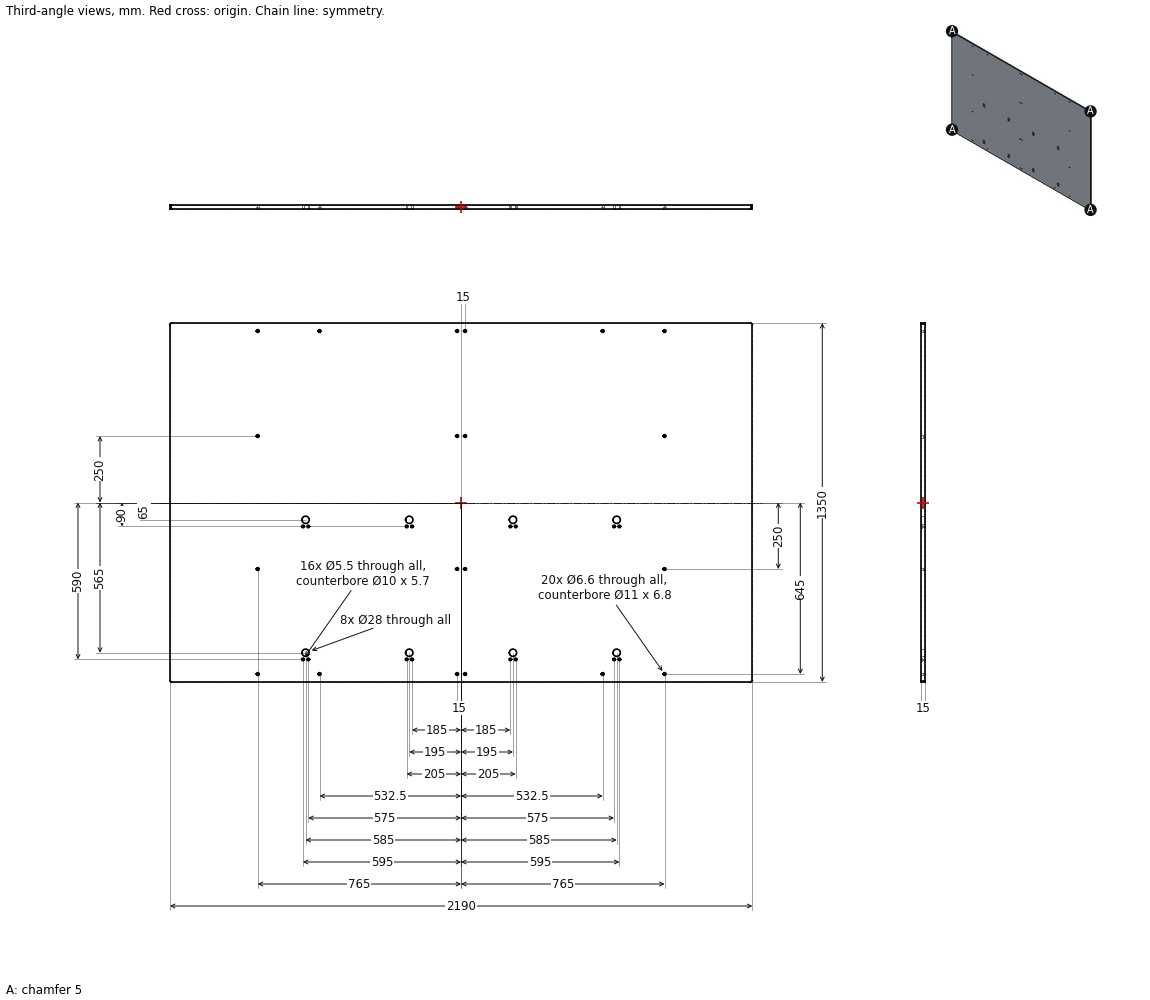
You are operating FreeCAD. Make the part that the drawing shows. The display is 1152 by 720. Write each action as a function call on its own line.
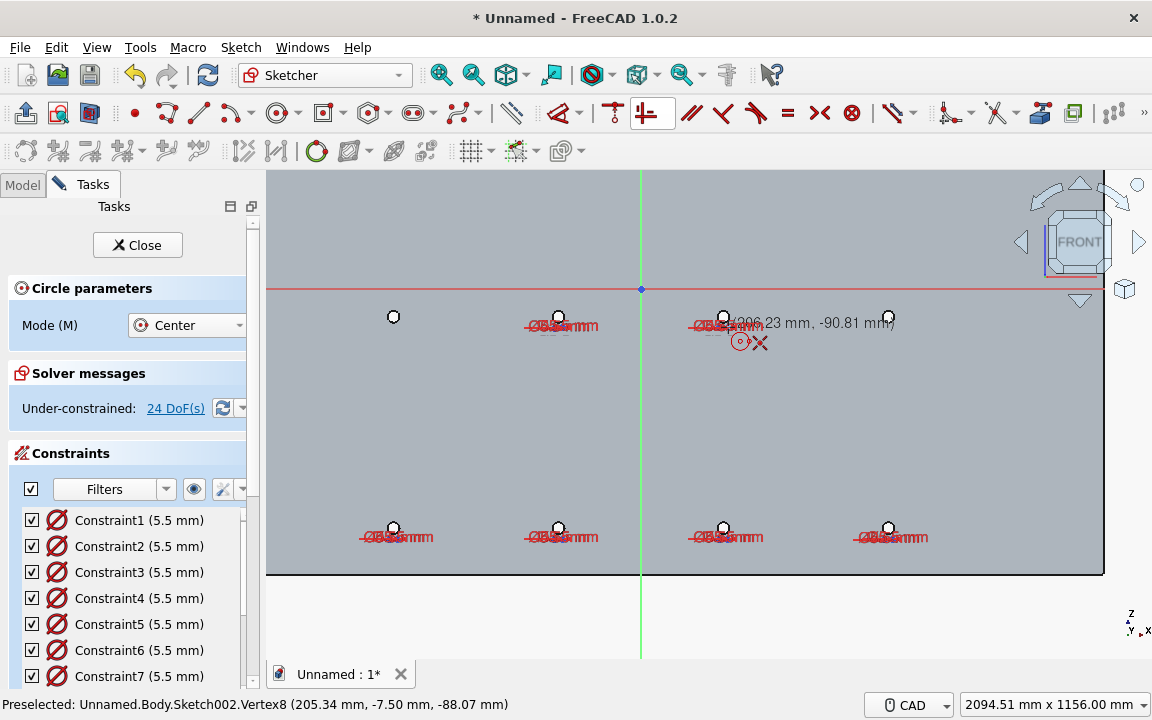
scroll(884, 327, up, 15)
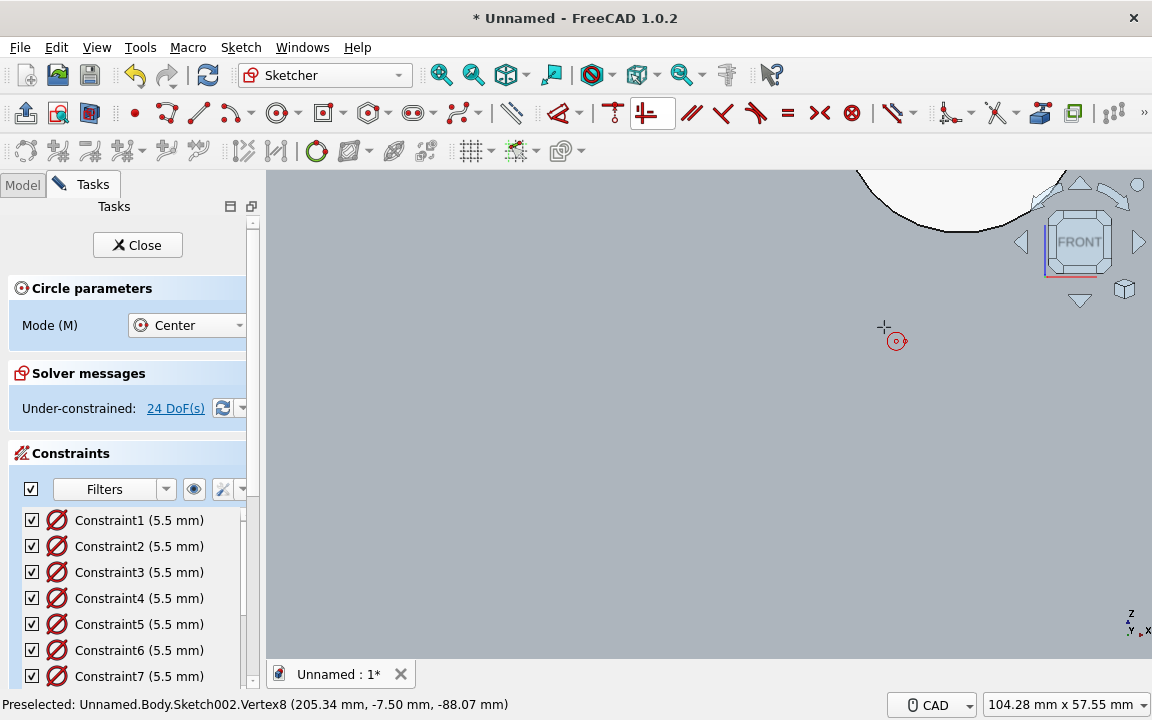
scroll(884, 327, down, 15)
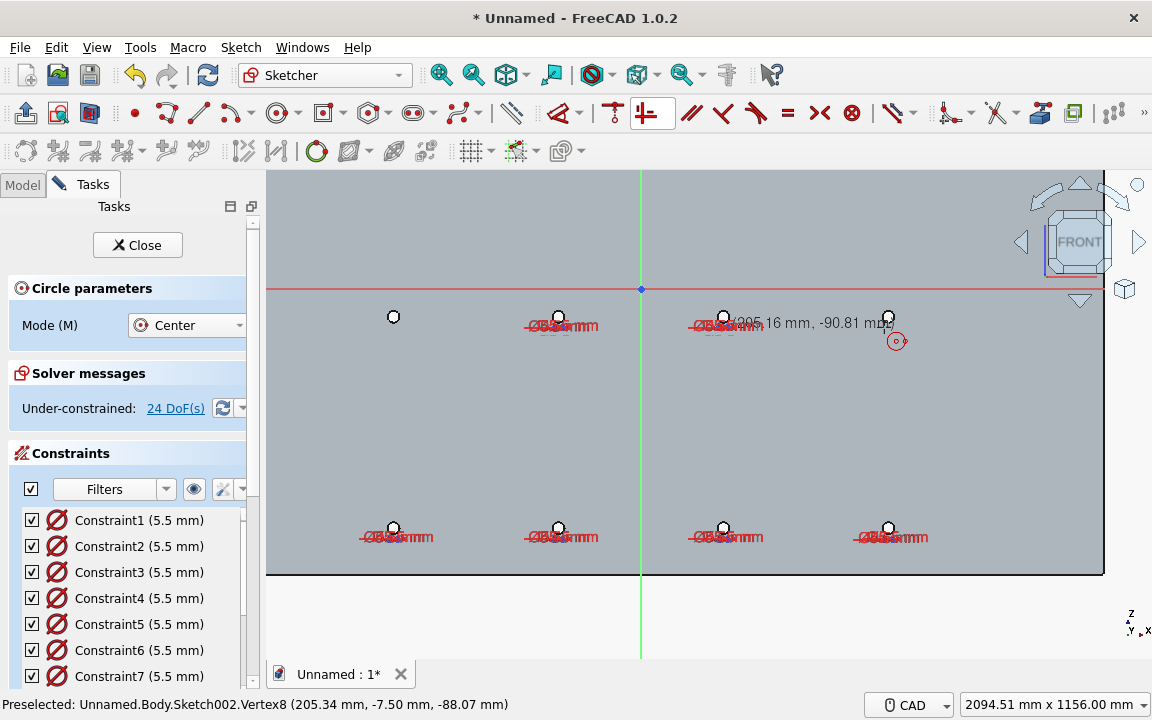
click(884, 327)
move(885, 326)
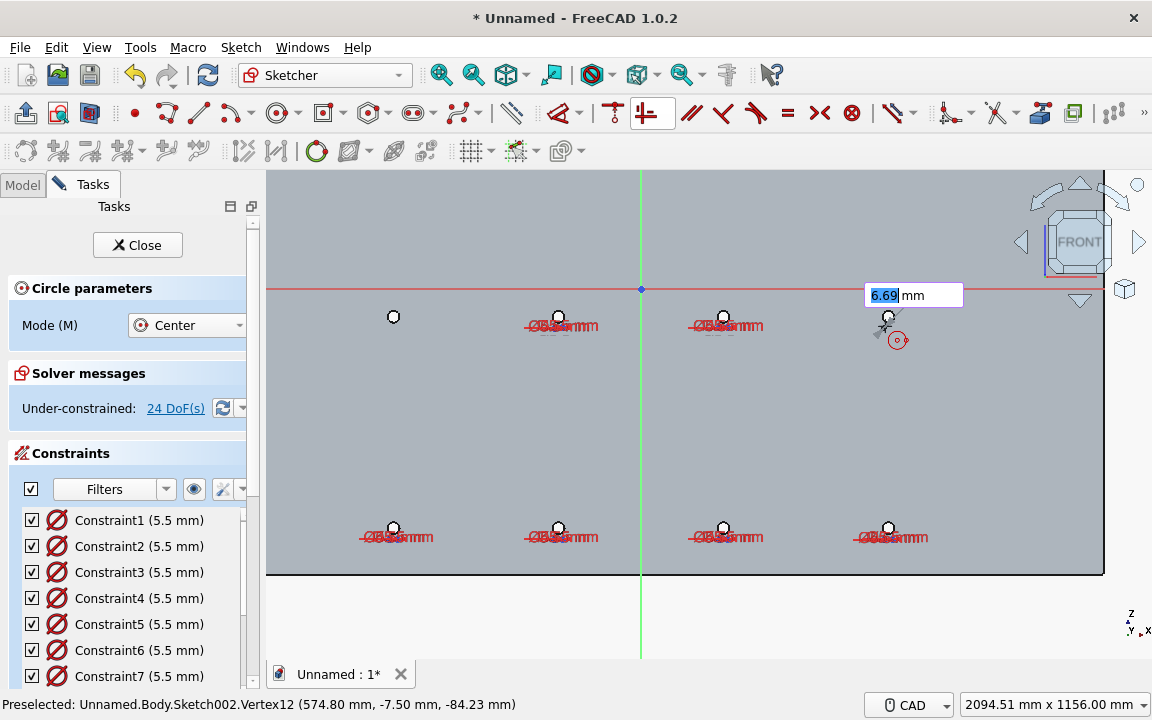
text(5.5)
key(Return)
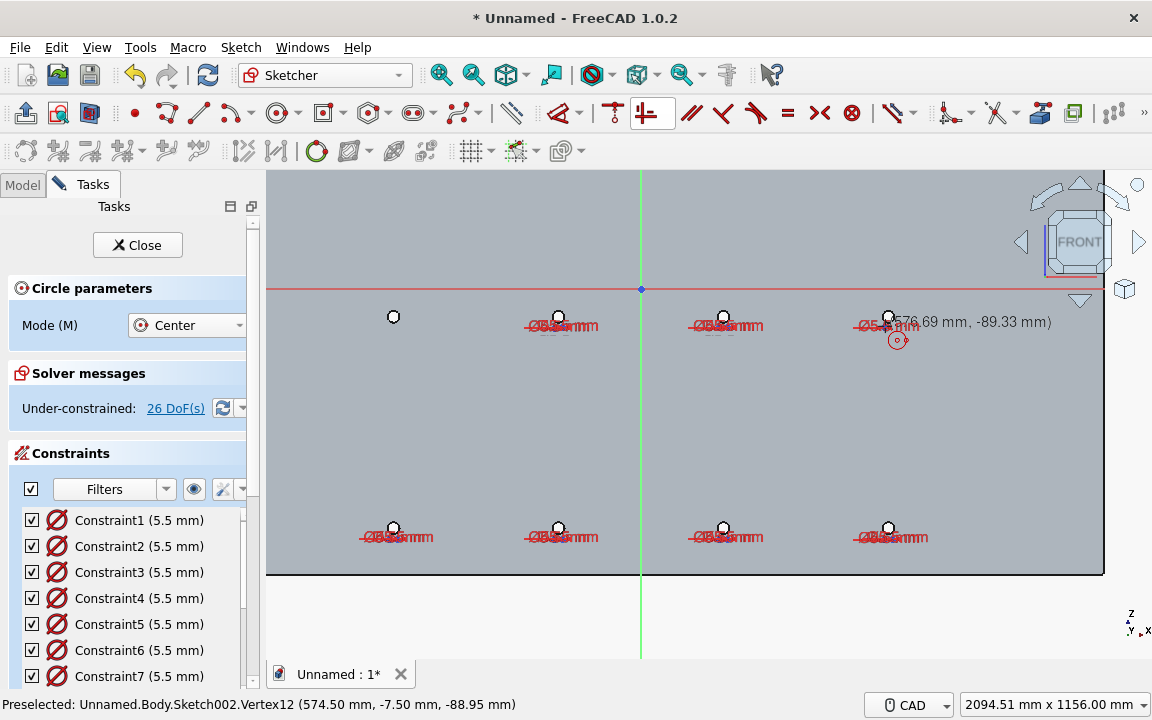
scroll(893, 327, up, 15)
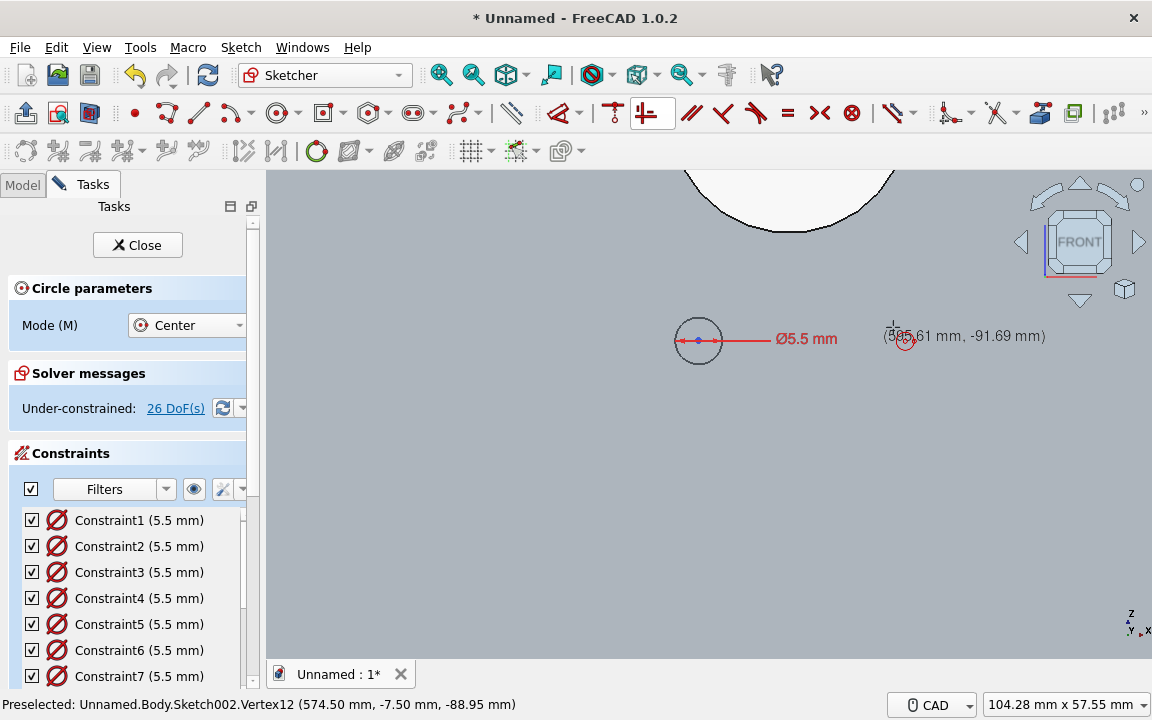
scroll(893, 327, down, 15)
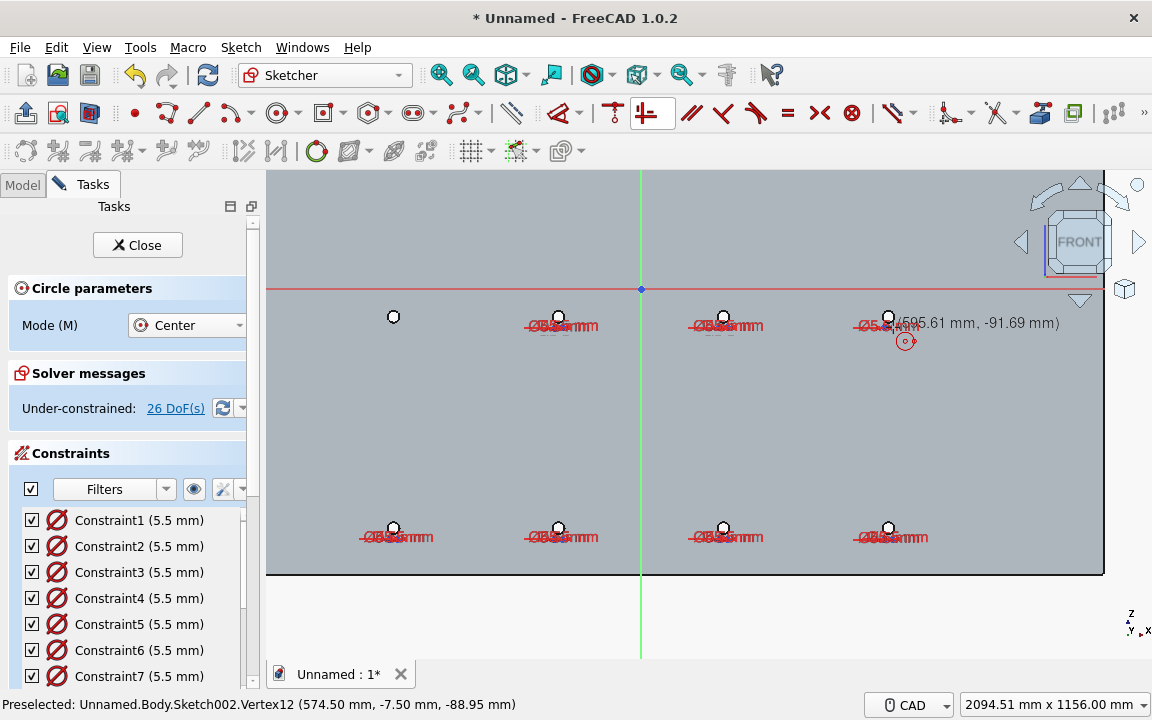
scroll(893, 327, up, 4)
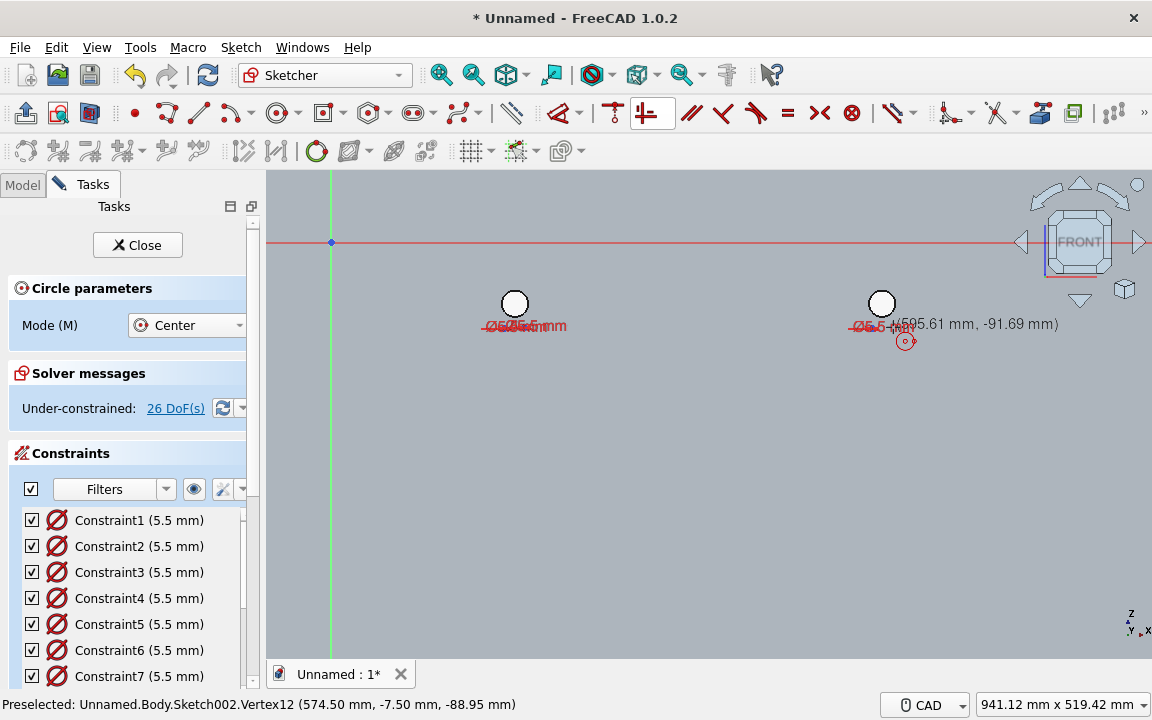
click(892, 327)
move(893, 325)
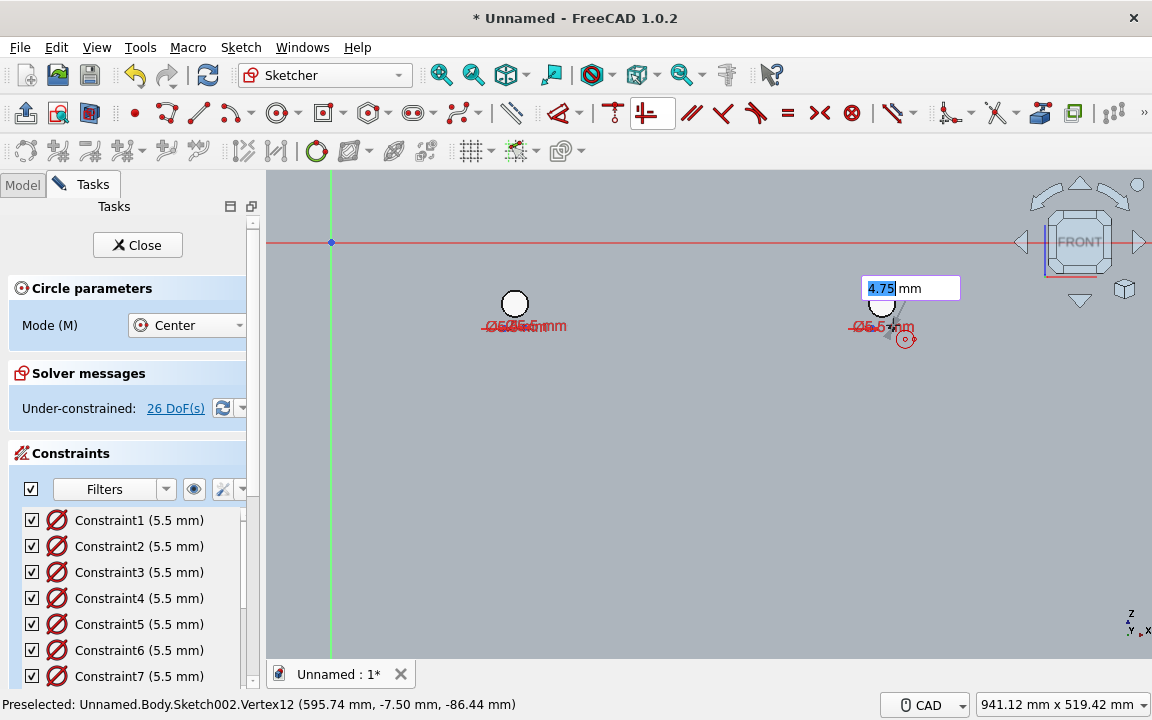
text(5.5)
key(Return)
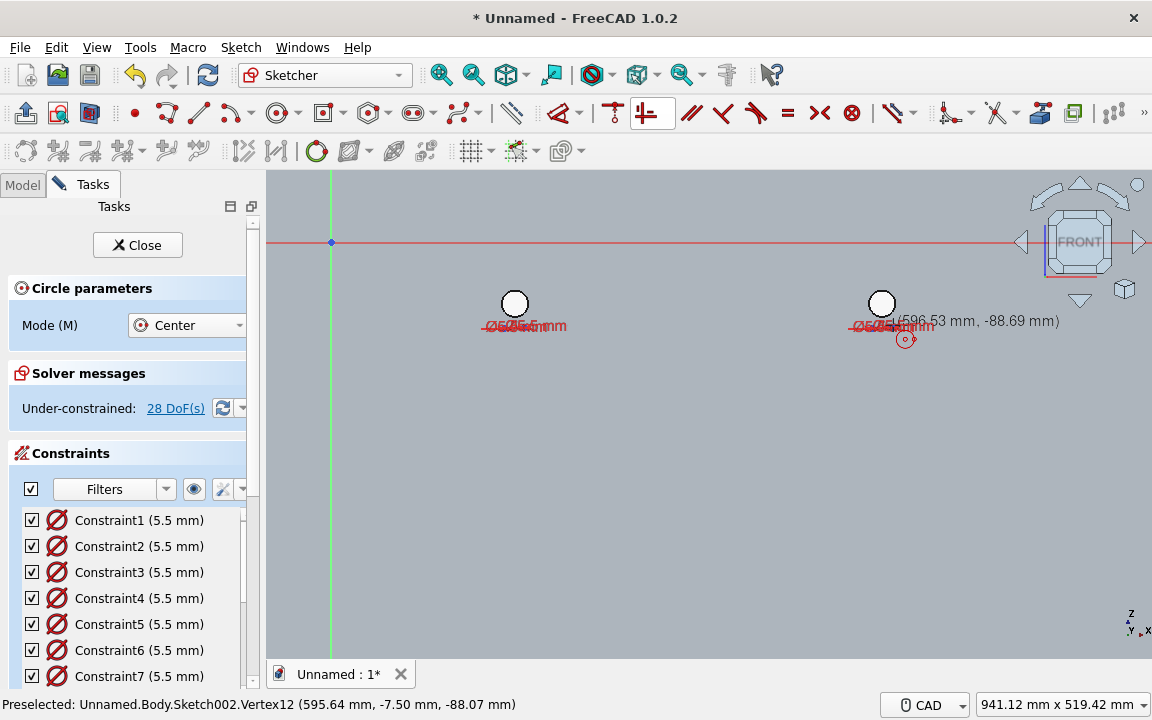
scroll(893, 327, down, 4)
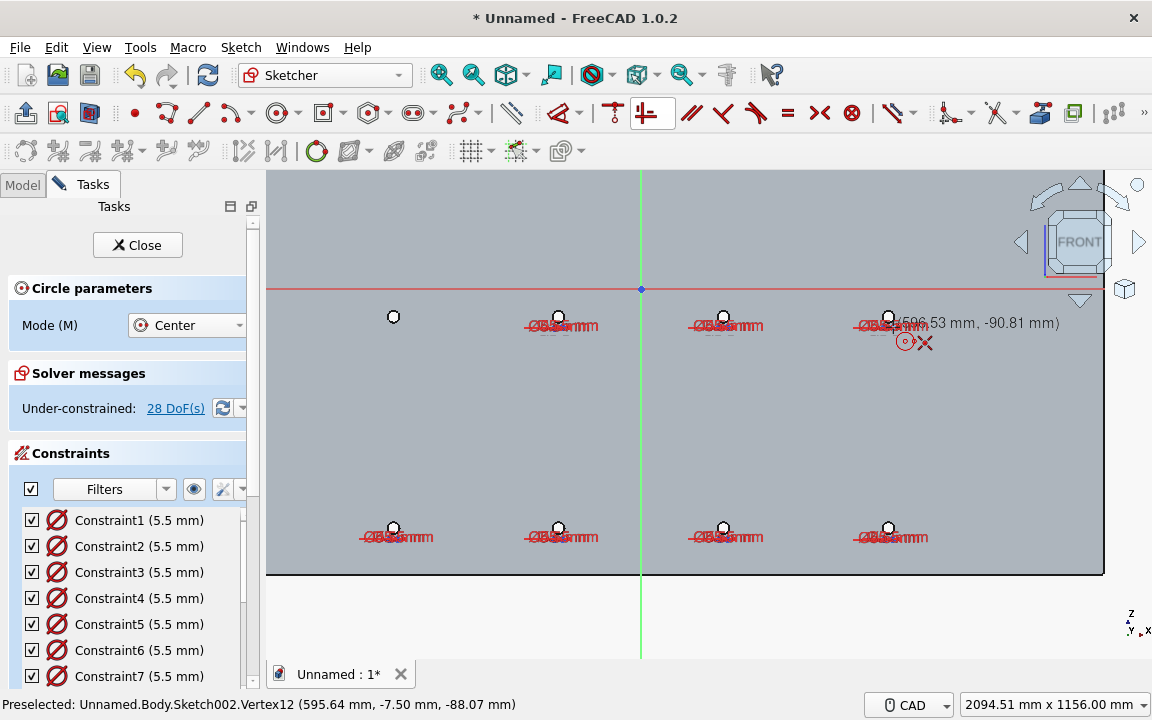
scroll(389, 327, up, 15)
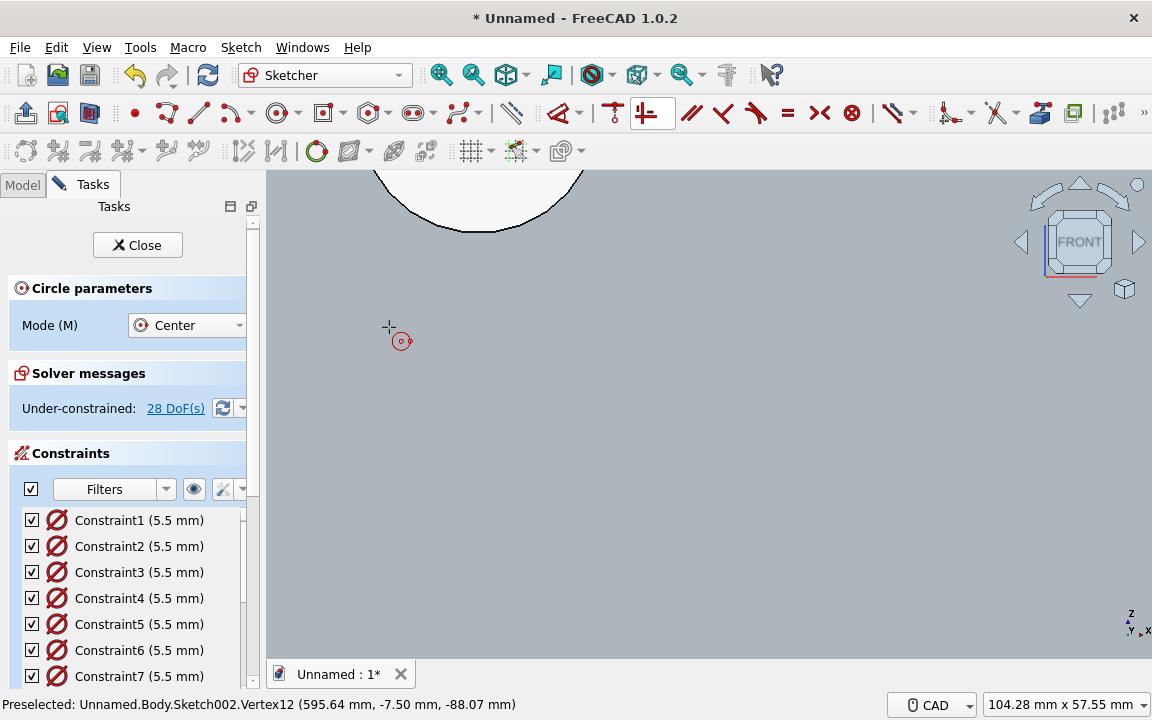
scroll(389, 327, down, 15)